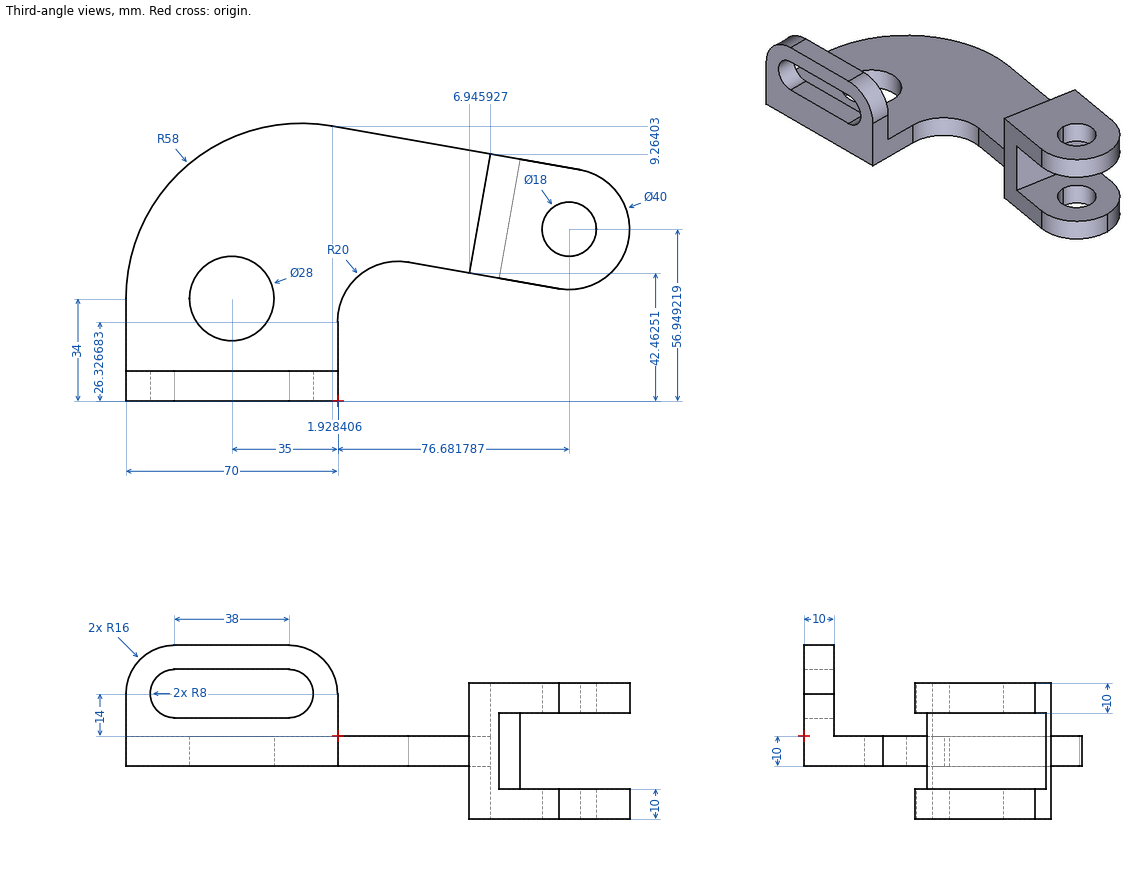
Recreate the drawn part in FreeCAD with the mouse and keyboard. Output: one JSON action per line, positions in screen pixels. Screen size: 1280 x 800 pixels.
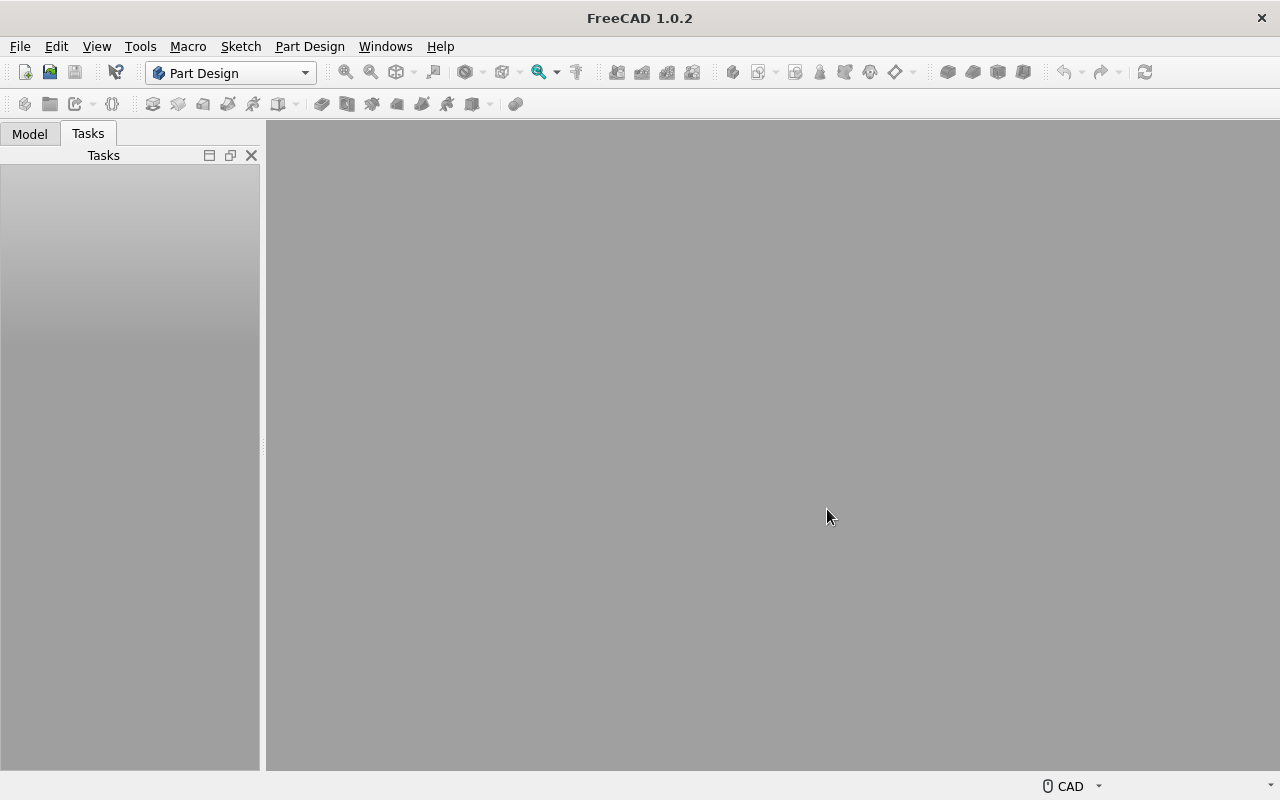
{"action": "left_click", "coordinate": [25, 72]}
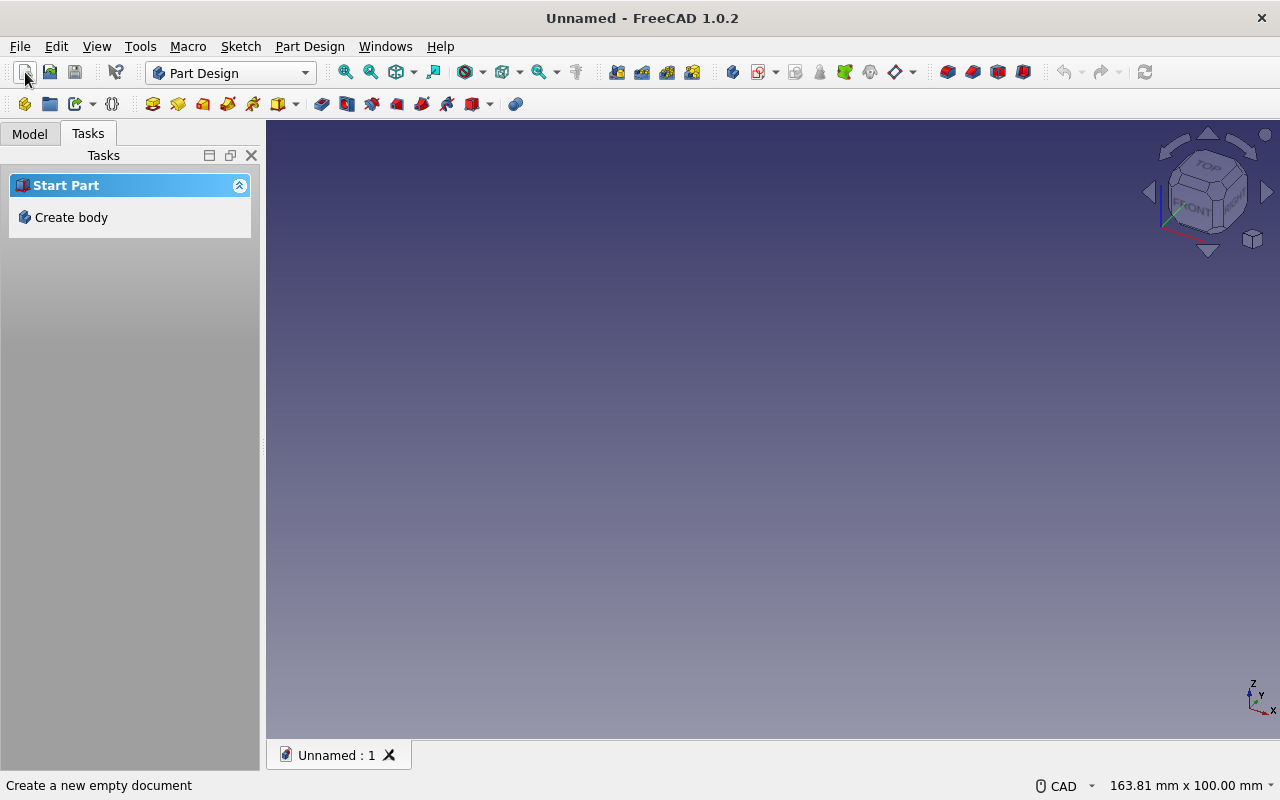
{"action": "left_click", "coordinate": [758, 72]}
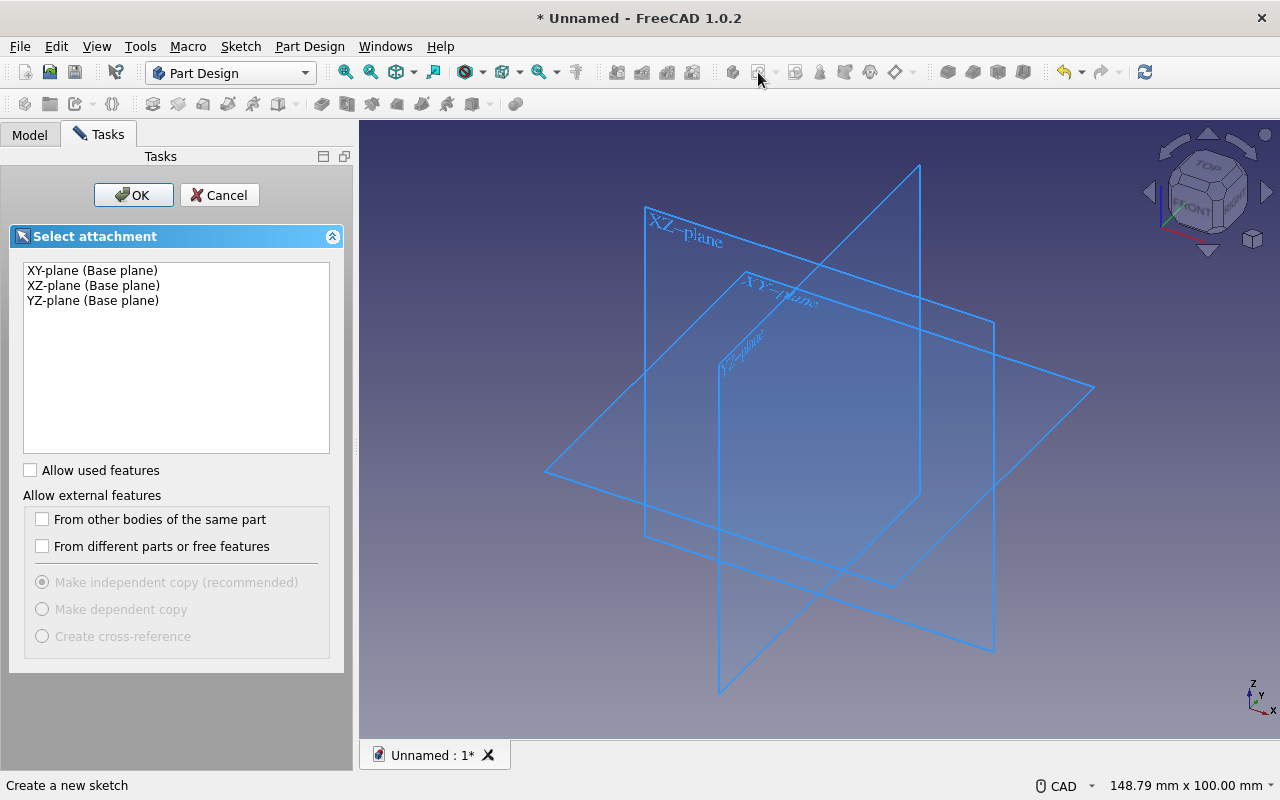
{"action": "left_click", "coordinate": [84, 286]}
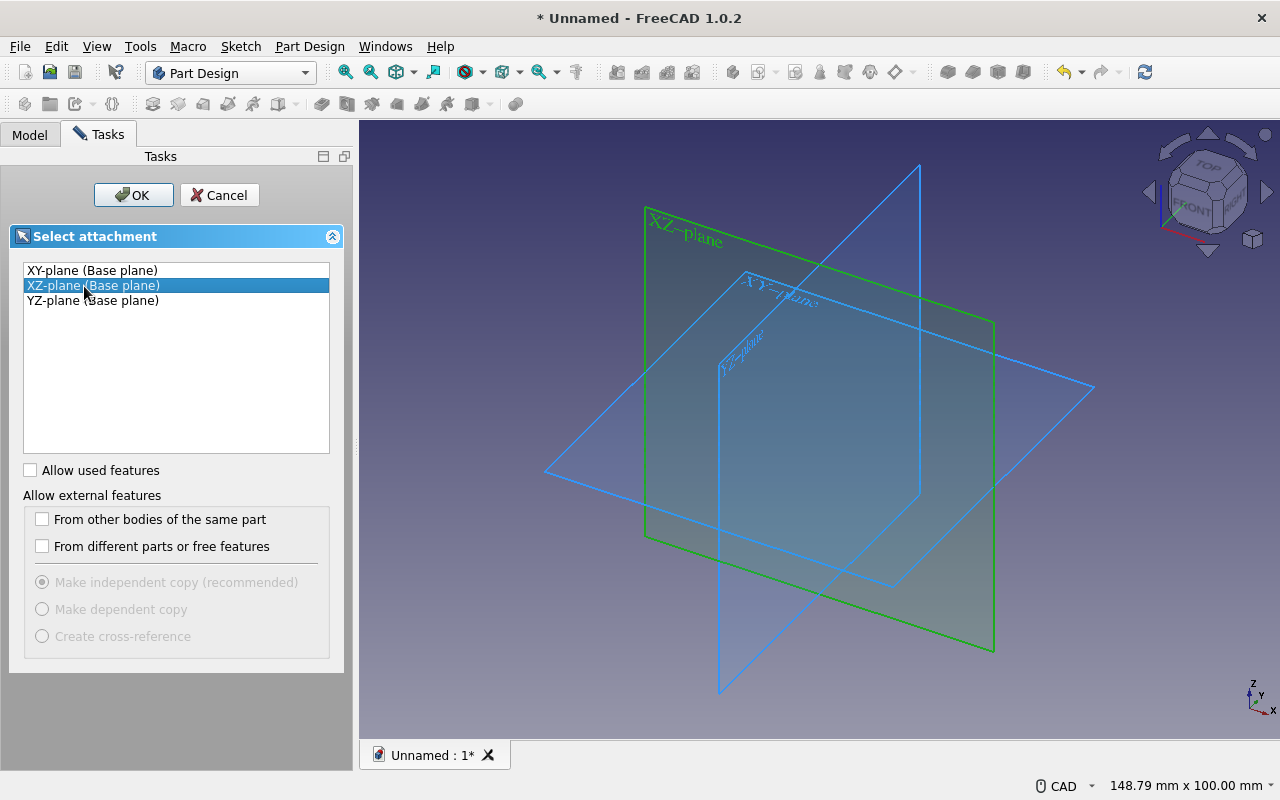
{"action": "left_click", "coordinate": [134, 195]}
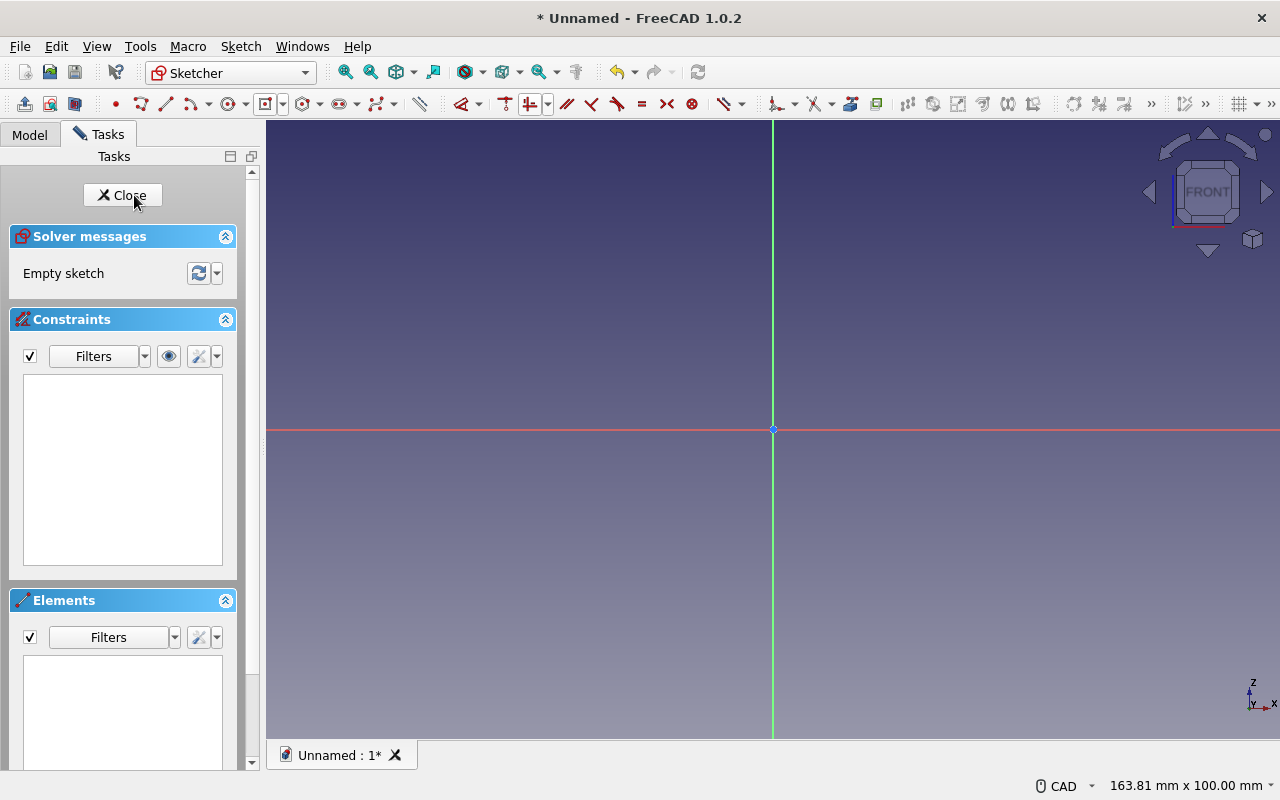
{"action": "left_click", "coordinate": [166, 104]}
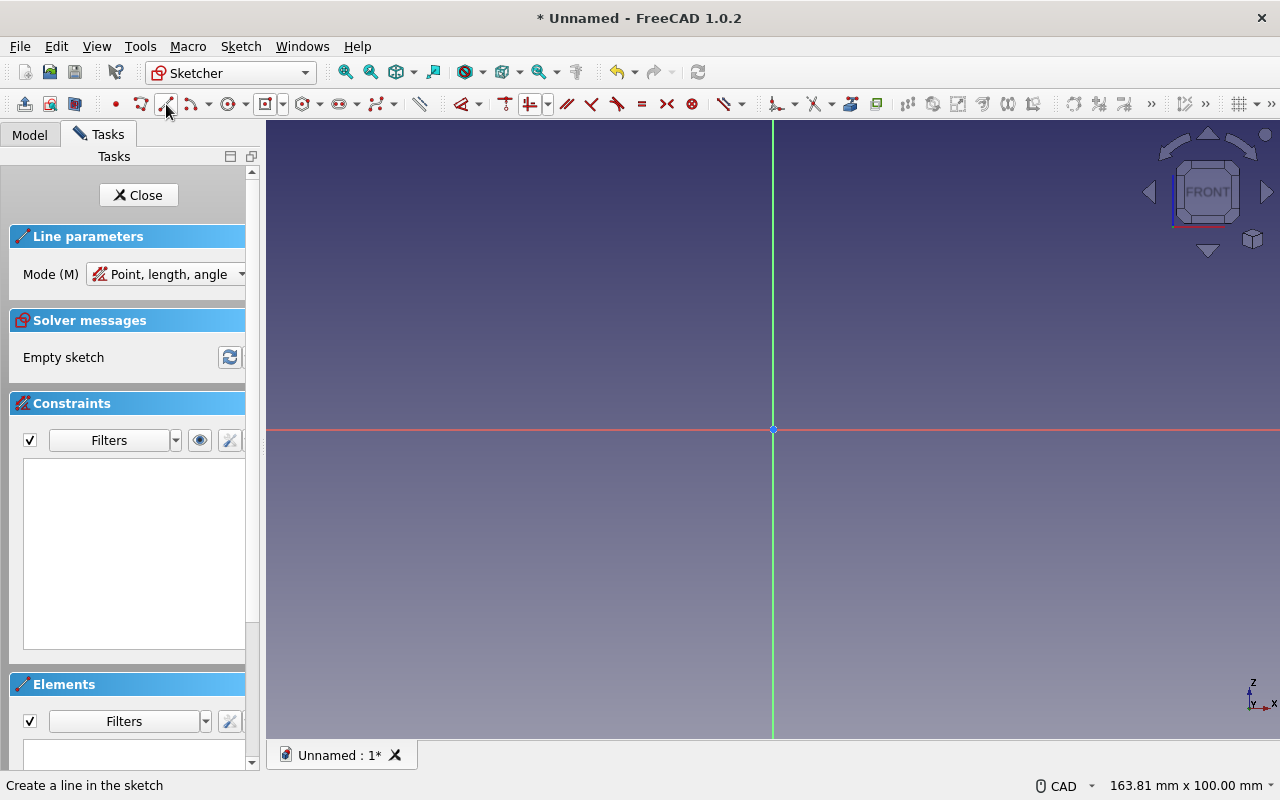
{"action": "left_click", "coordinate": [439, 244]}
{"action": "left_click", "coordinate": [674, 244]}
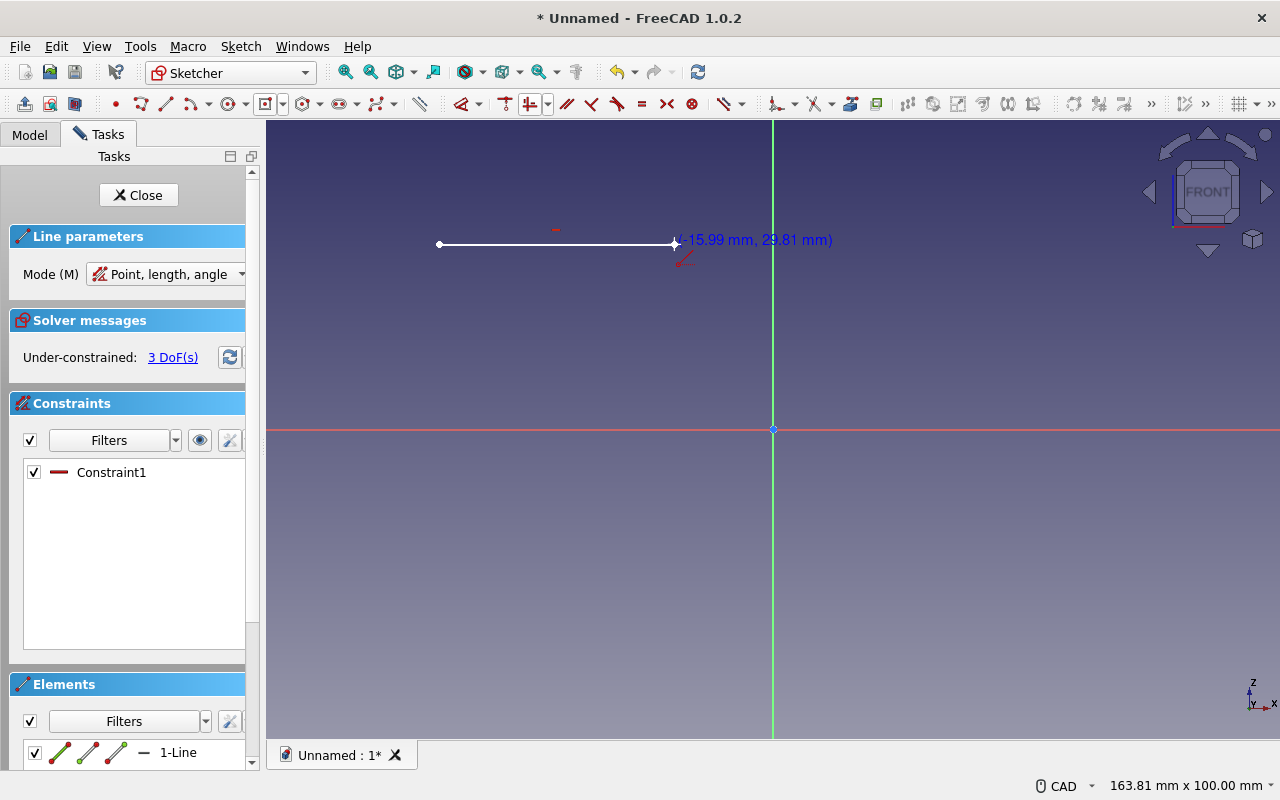
{"action": "left_click", "coordinate": [141, 104]}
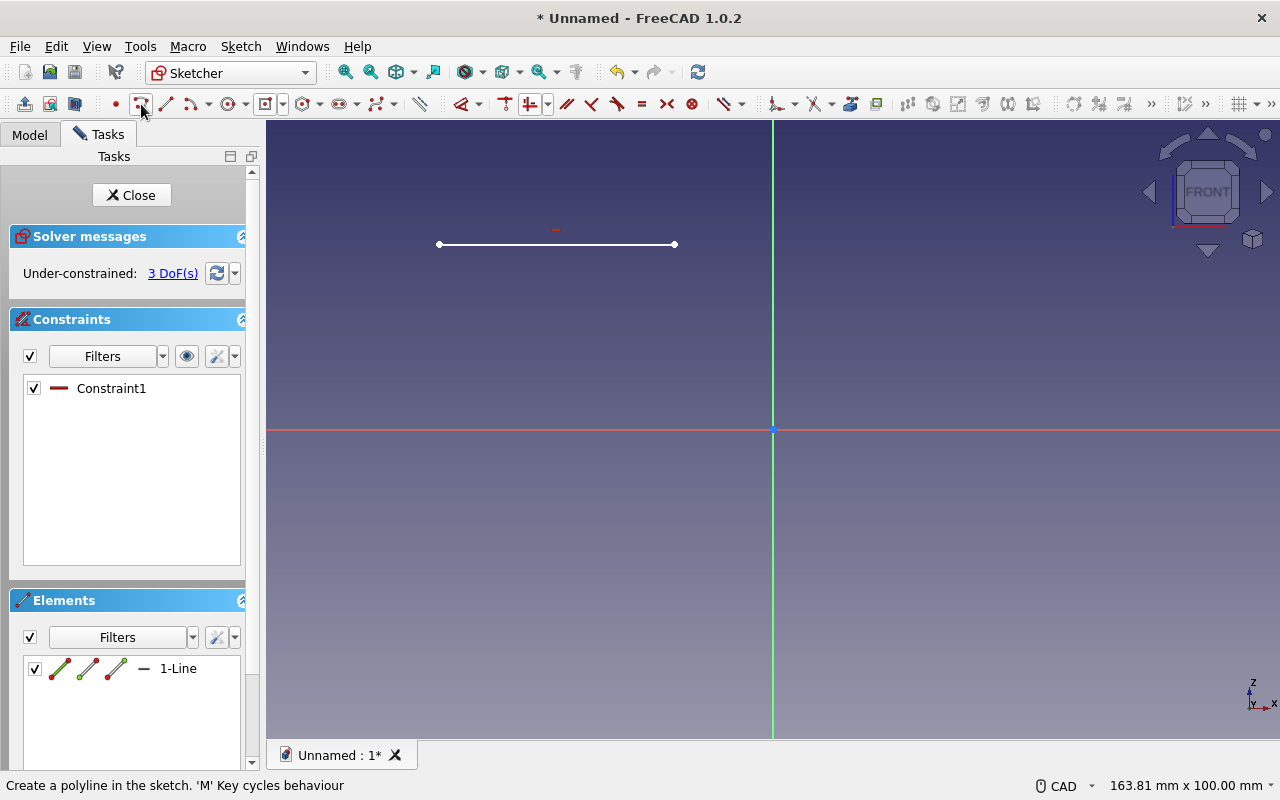
{"action": "left_click", "coordinate": [773, 343]}
{"action": "left_click", "coordinate": [773, 430]}
{"action": "left_click", "coordinate": [340, 420]}
{"action": "left_click", "coordinate": [340, 343]}
{"action": "right_click", "coordinate": [340, 343]}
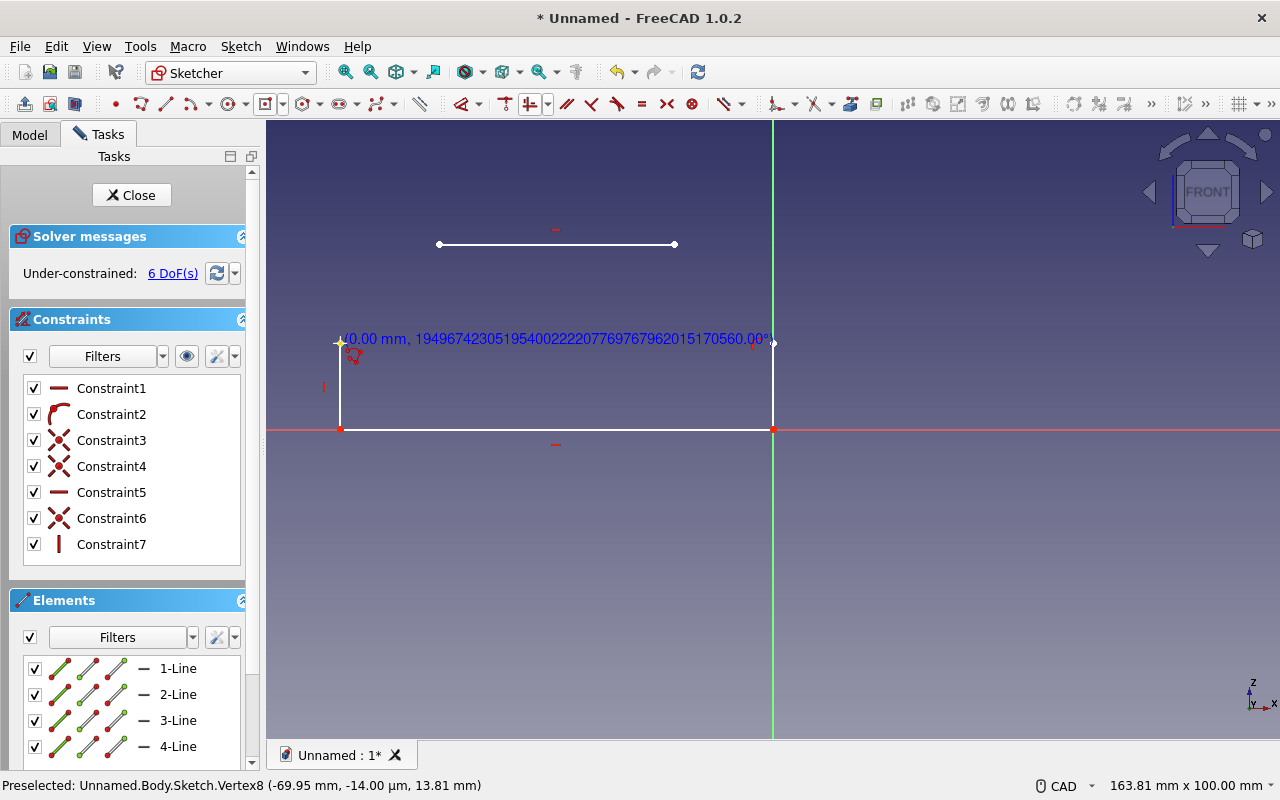
{"action": "left_click", "coordinate": [208, 104]}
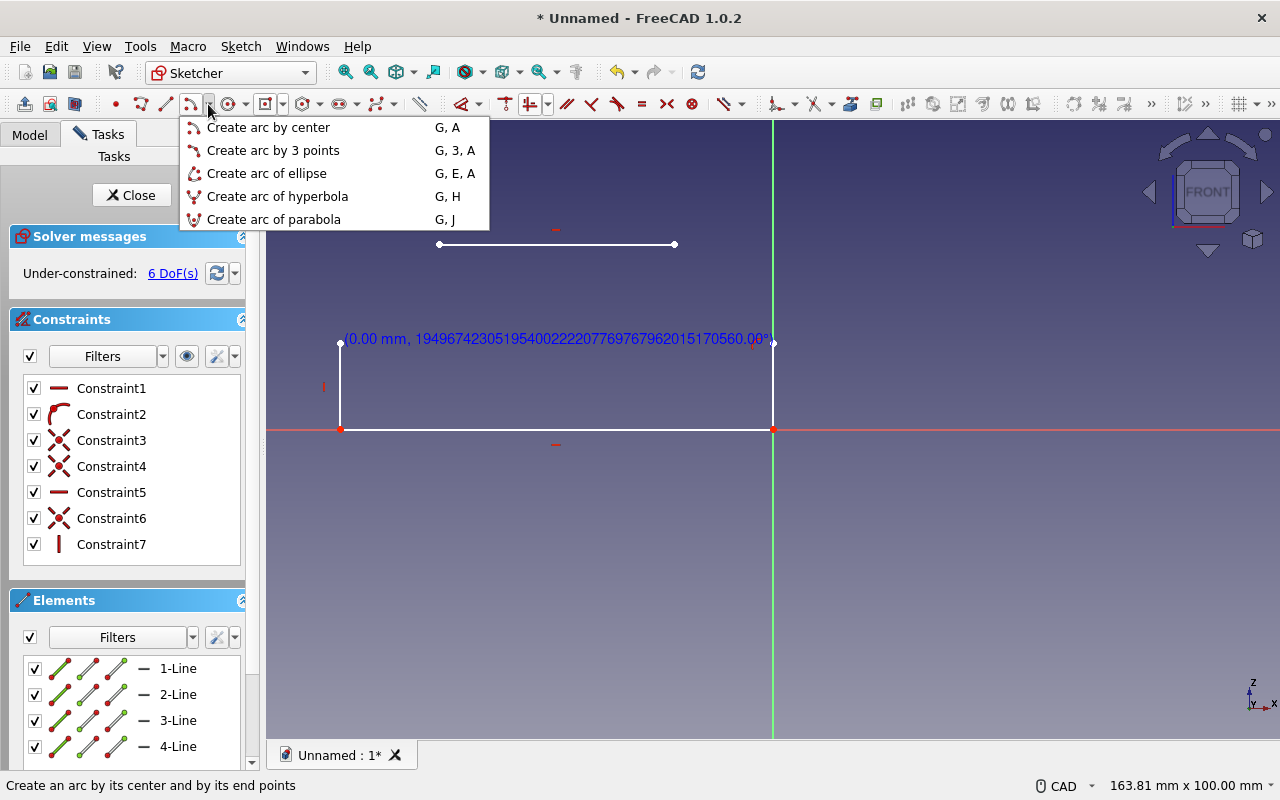
{"action": "left_click", "coordinate": [334, 150]}